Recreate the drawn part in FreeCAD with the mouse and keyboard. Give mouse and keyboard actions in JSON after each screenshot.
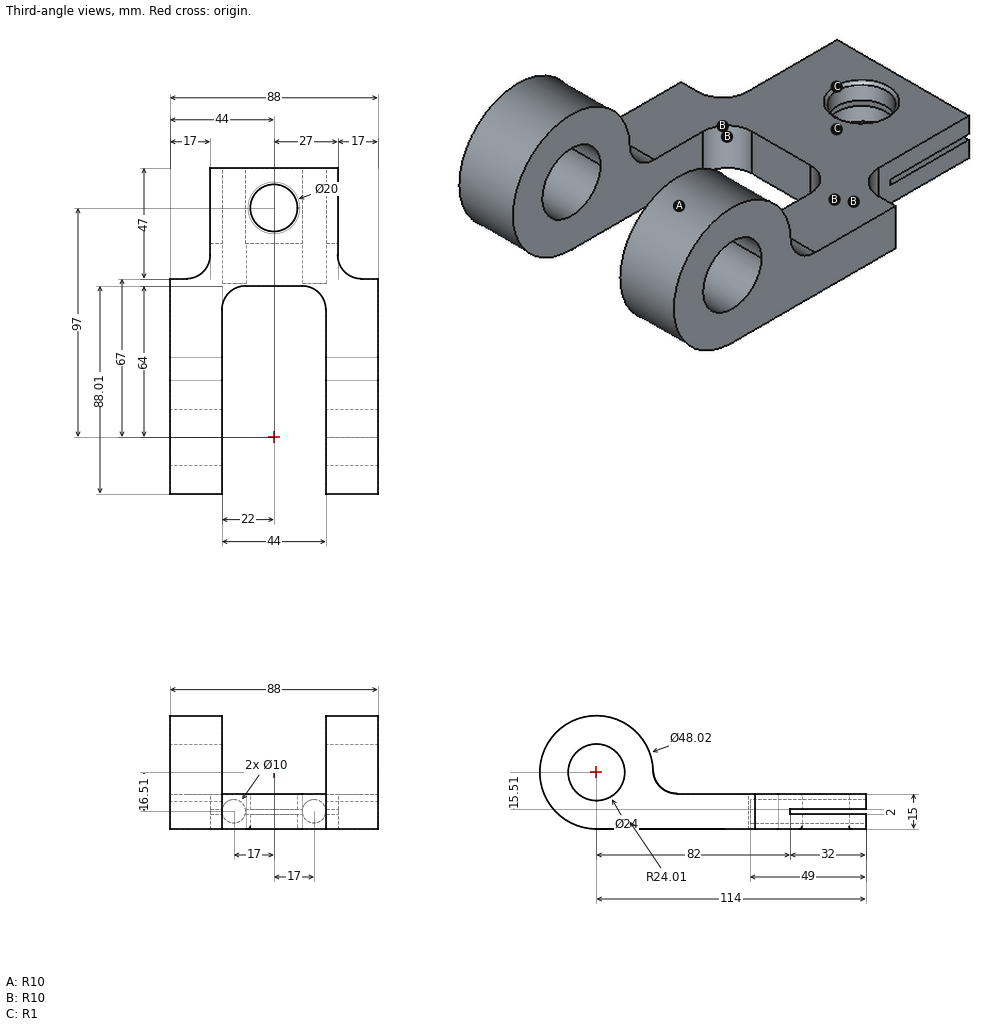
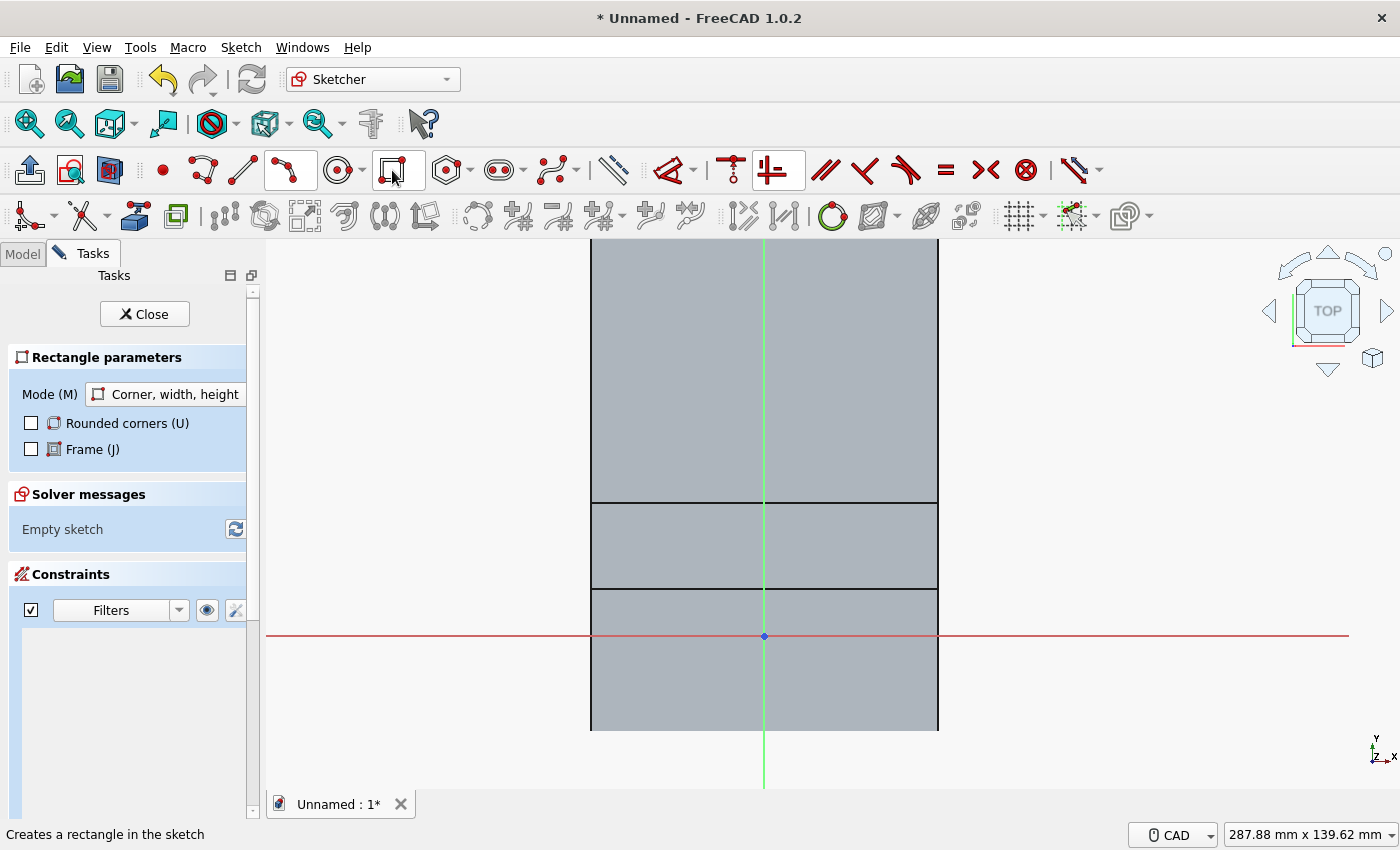
{"action": "left_click", "coordinate": [678, 384]}
{"action": "left_click", "coordinate": [851, 731]}
{"action": "key", "text": "Escape"}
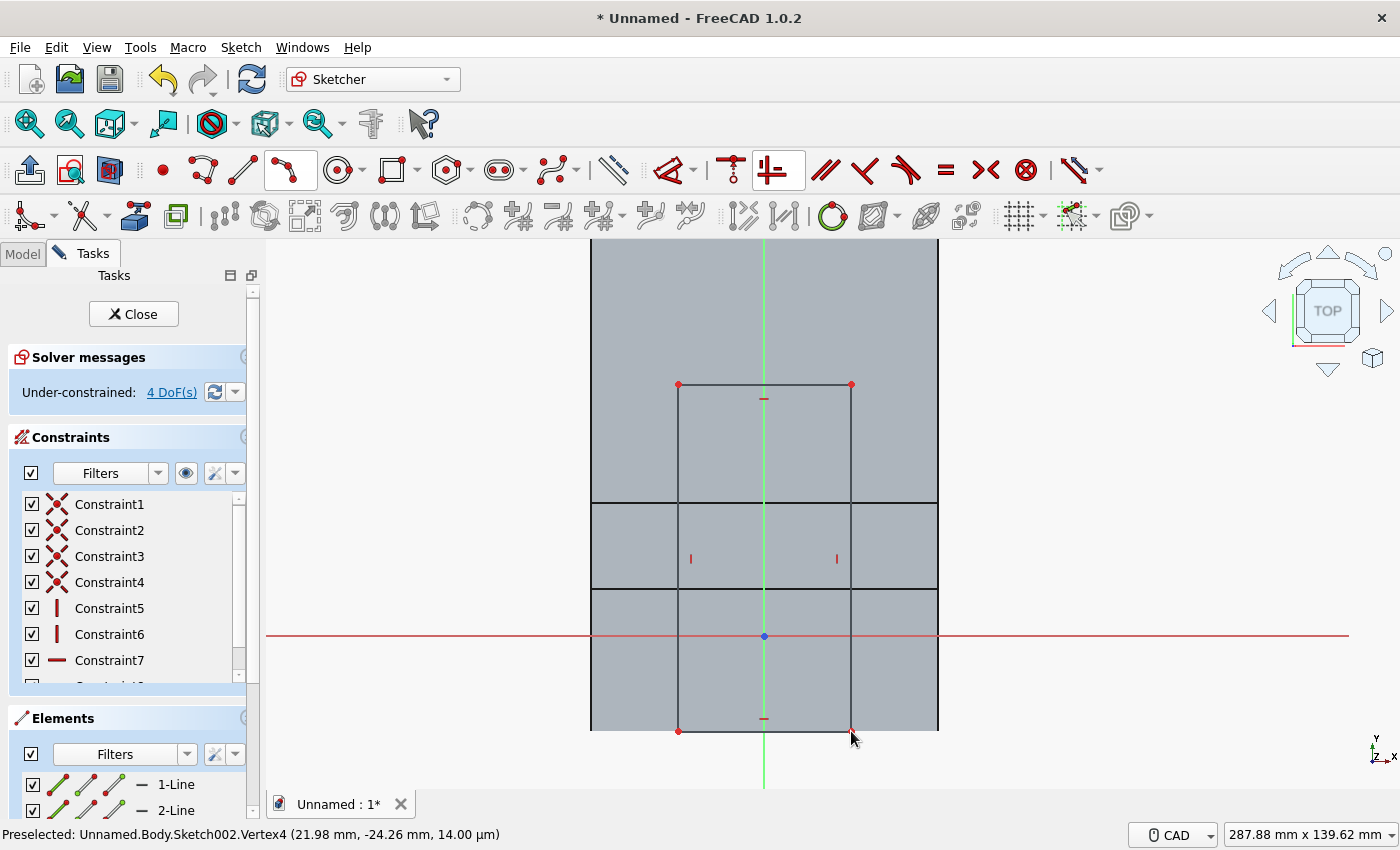
{"action": "left_click", "coordinate": [668, 170]}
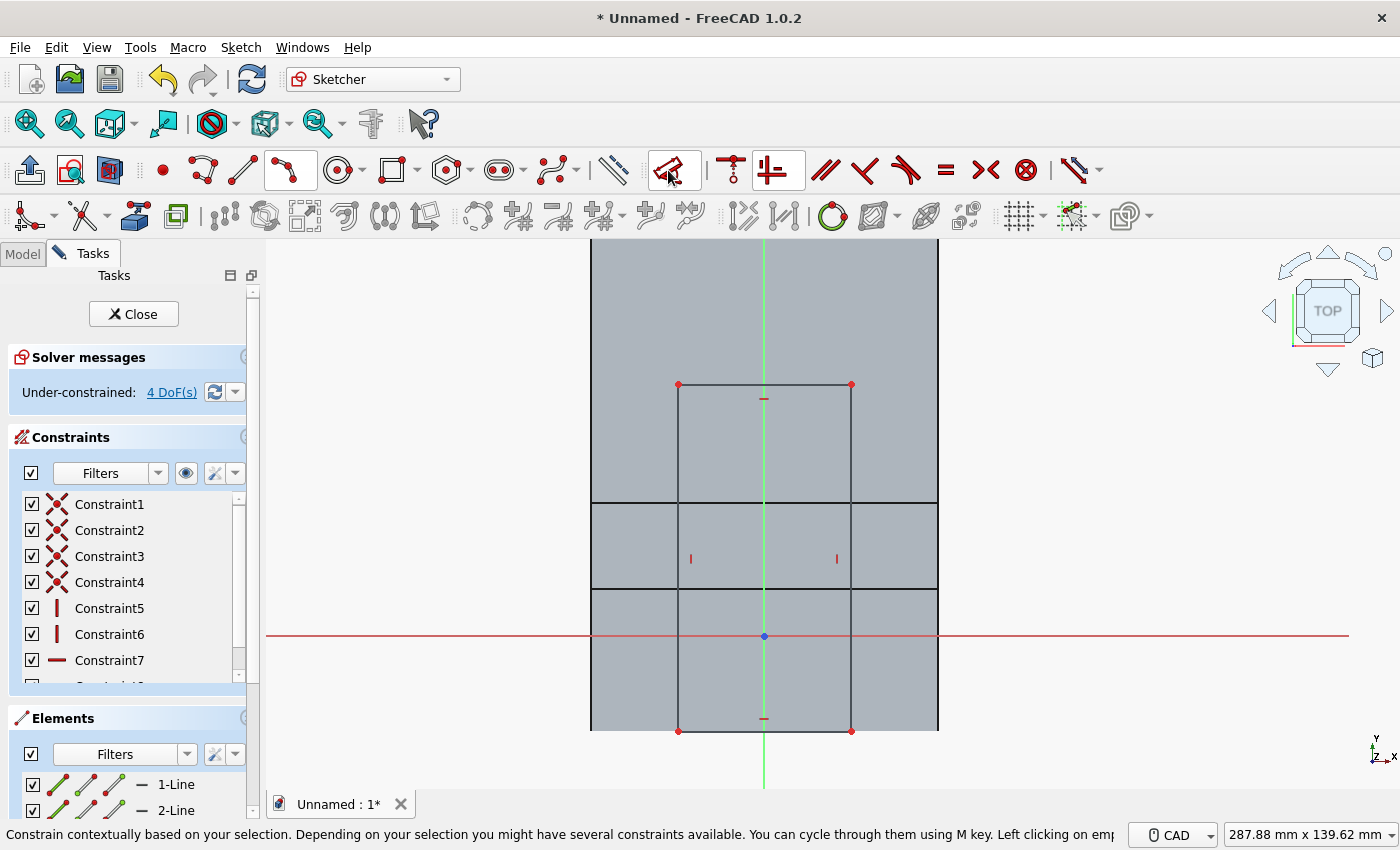
{"action": "left_click", "coordinate": [730, 732]}
{"action": "left_click", "coordinate": [725, 698]}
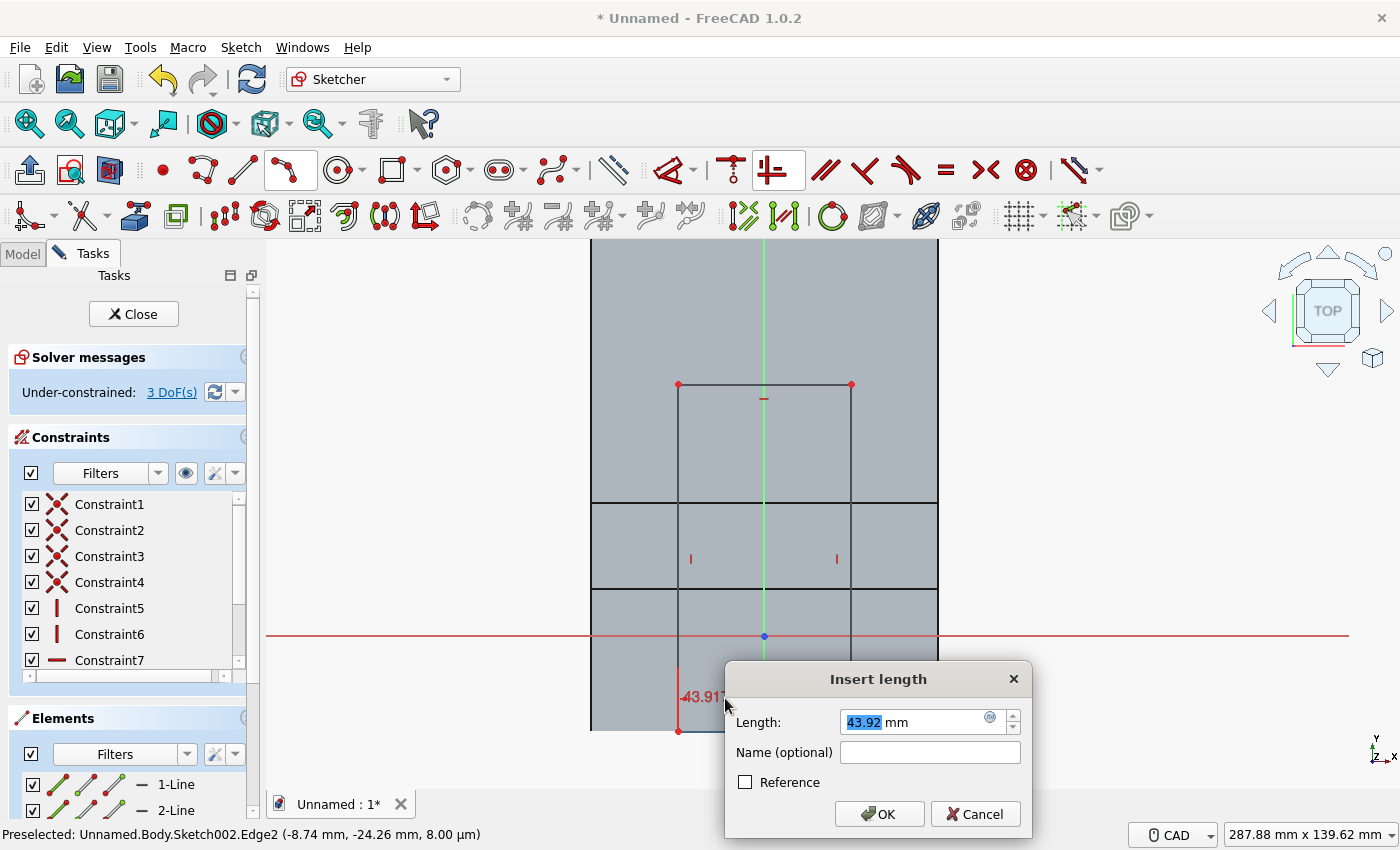
{"action": "type", "text": "44"}
{"action": "key", "text": "Return"}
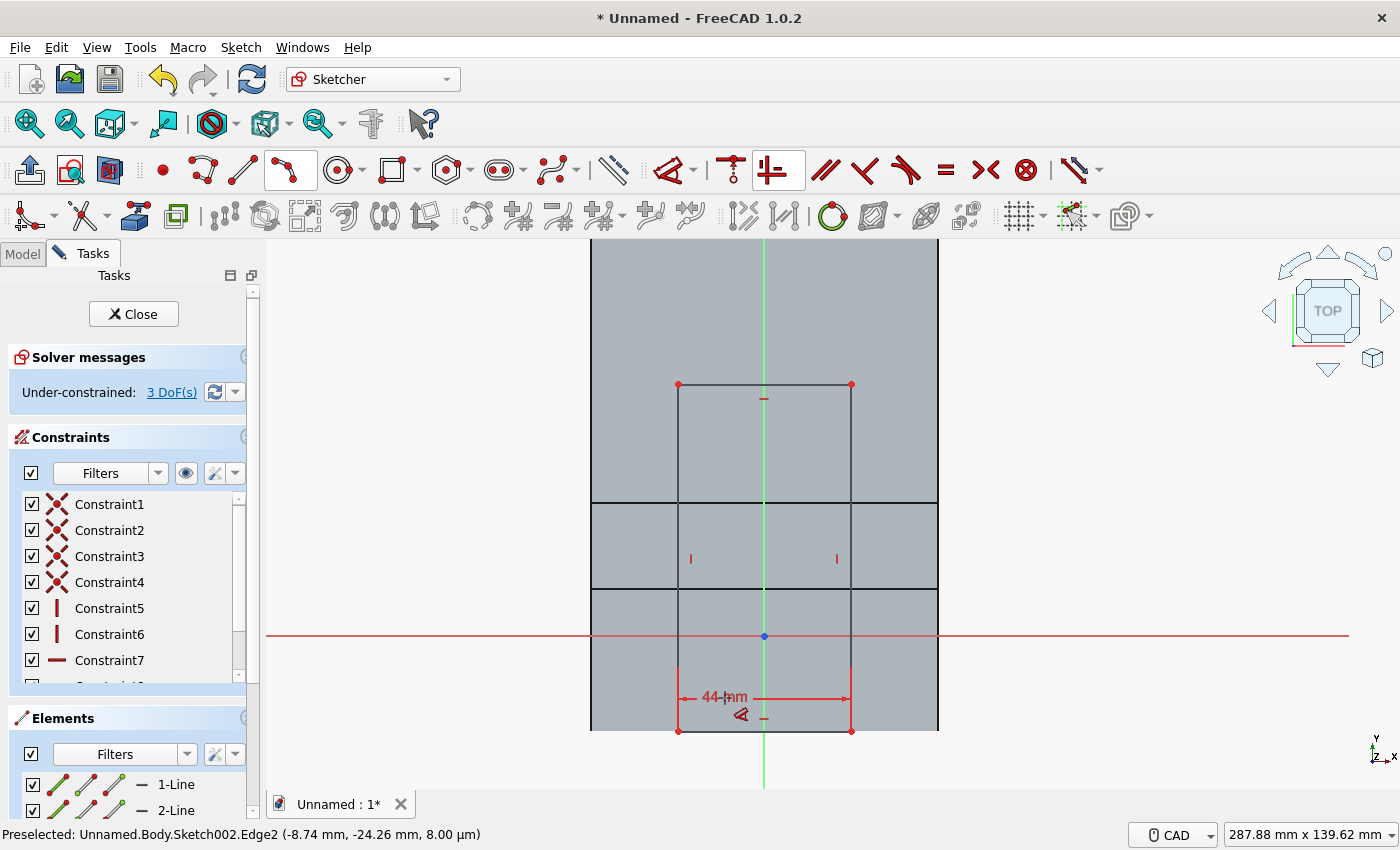
{"action": "left_click", "coordinate": [678, 385]}
{"action": "left_click", "coordinate": [721, 351]}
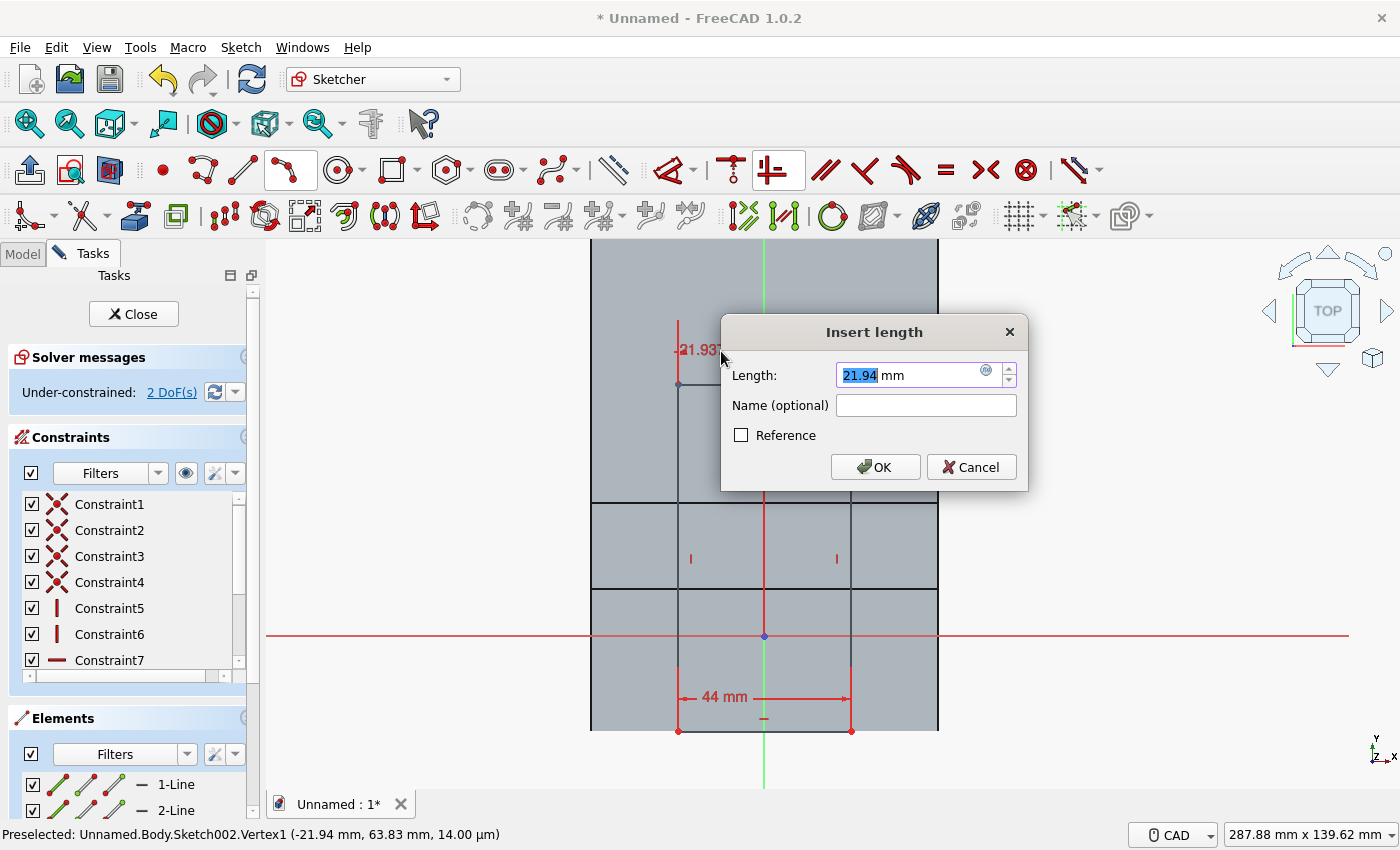
{"action": "type", "text": "22"}
{"action": "key", "text": "Return"}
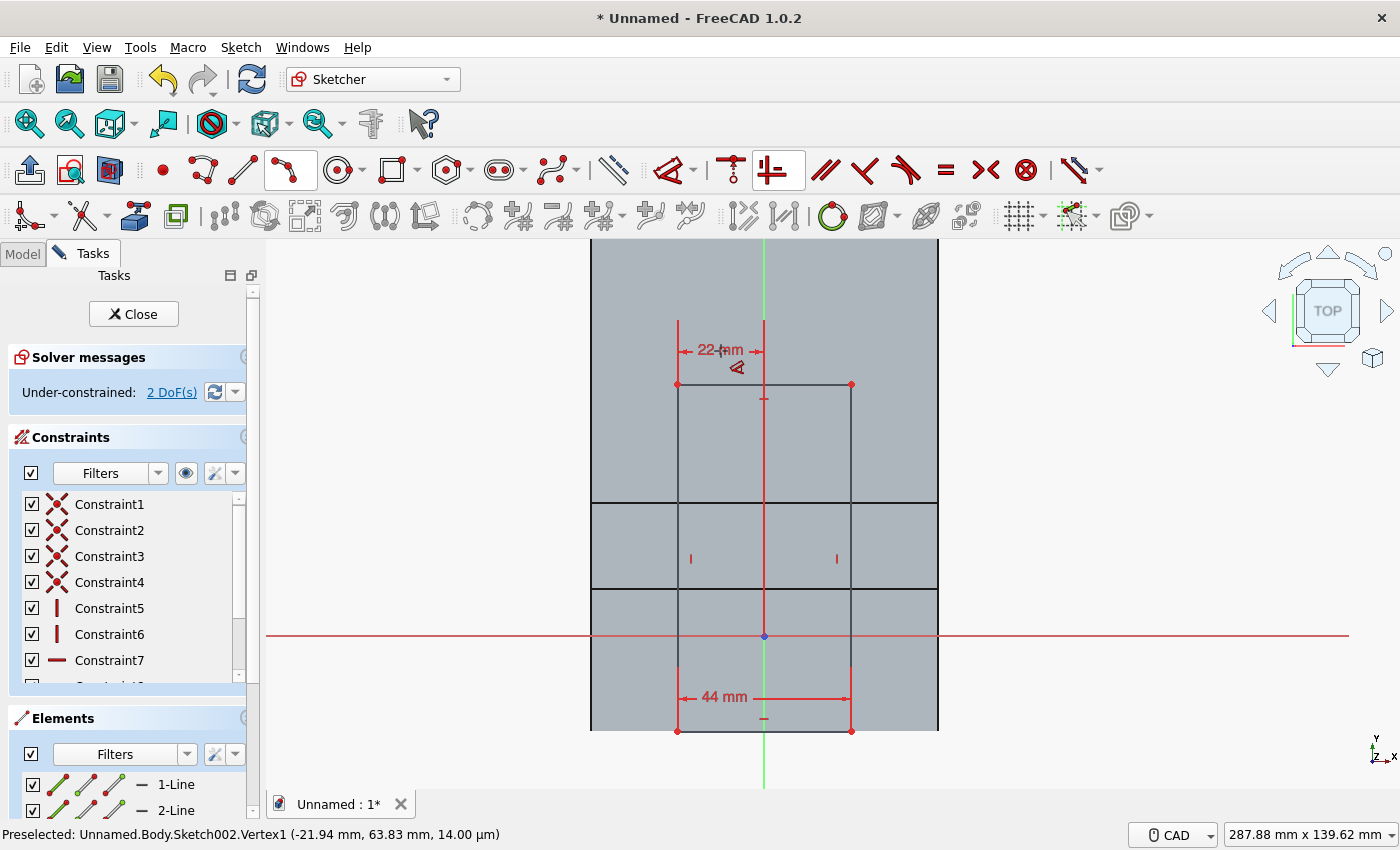
{"action": "left_click", "coordinate": [678, 385]}
{"action": "left_click", "coordinate": [644, 511]}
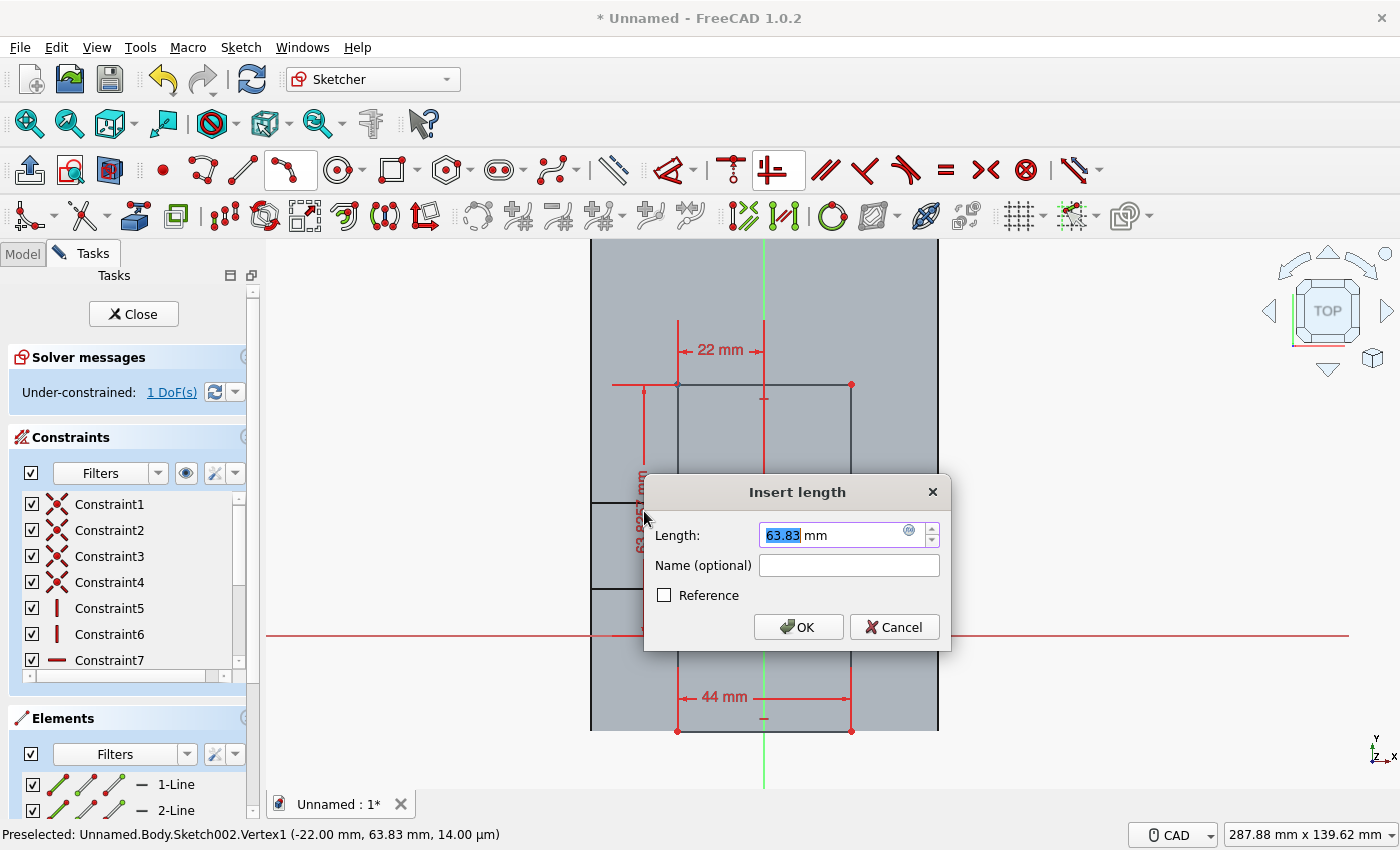
{"action": "type", "text": "64"}
{"action": "key", "text": "Return"}